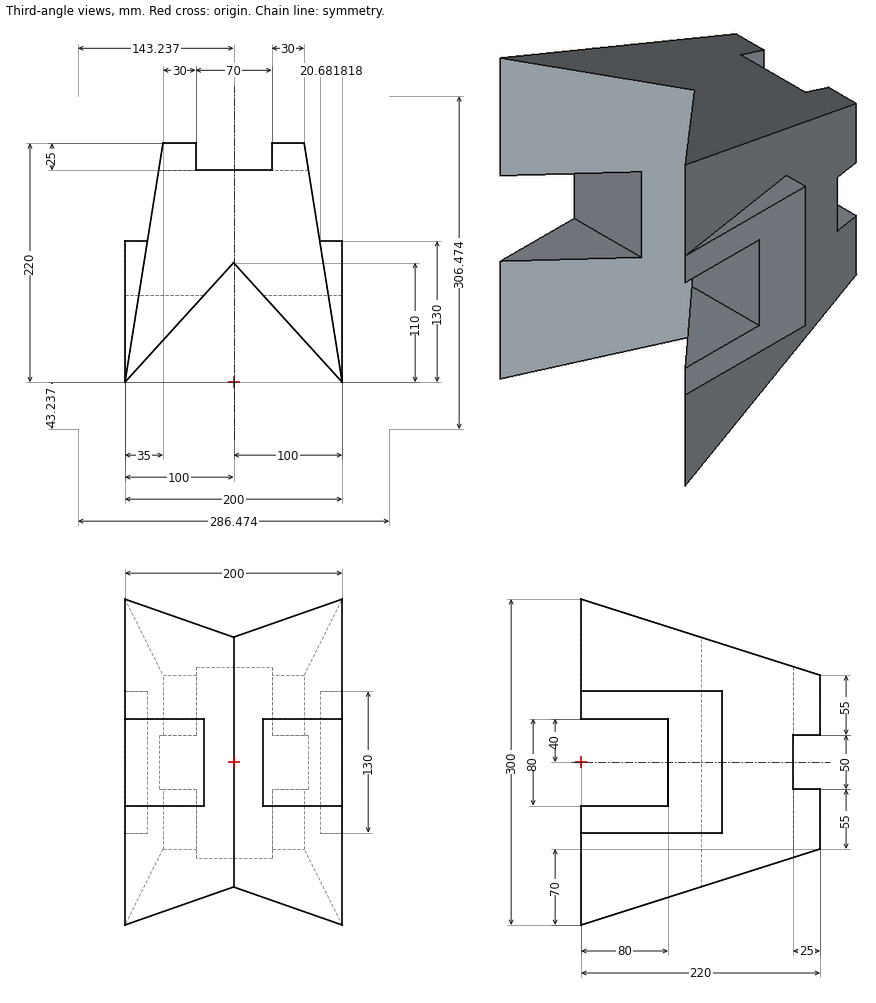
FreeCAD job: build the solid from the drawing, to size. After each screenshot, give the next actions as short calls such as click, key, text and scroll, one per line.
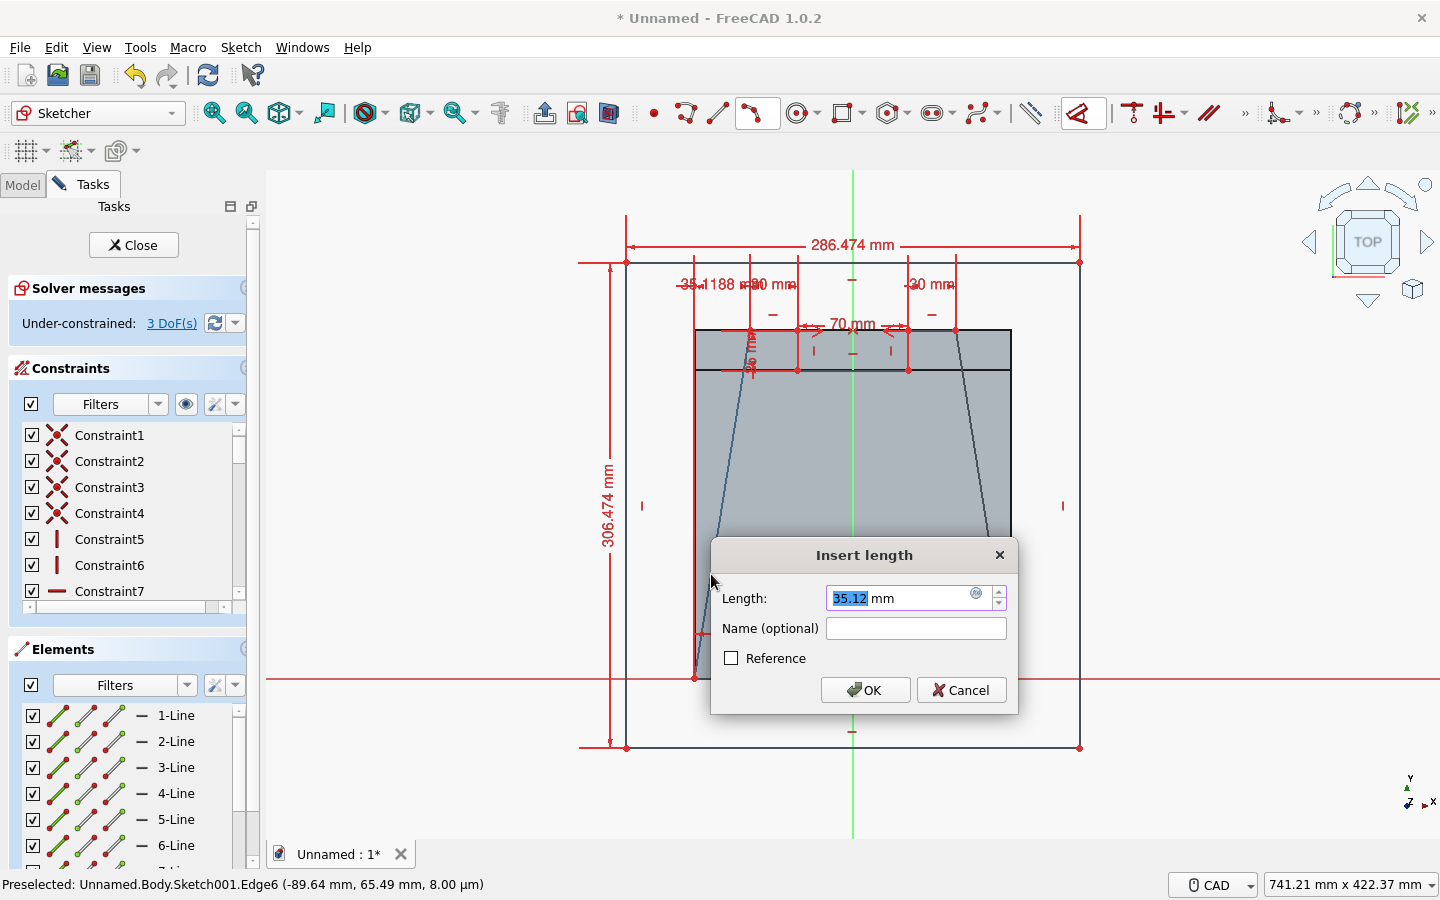
text(35)
key(Return)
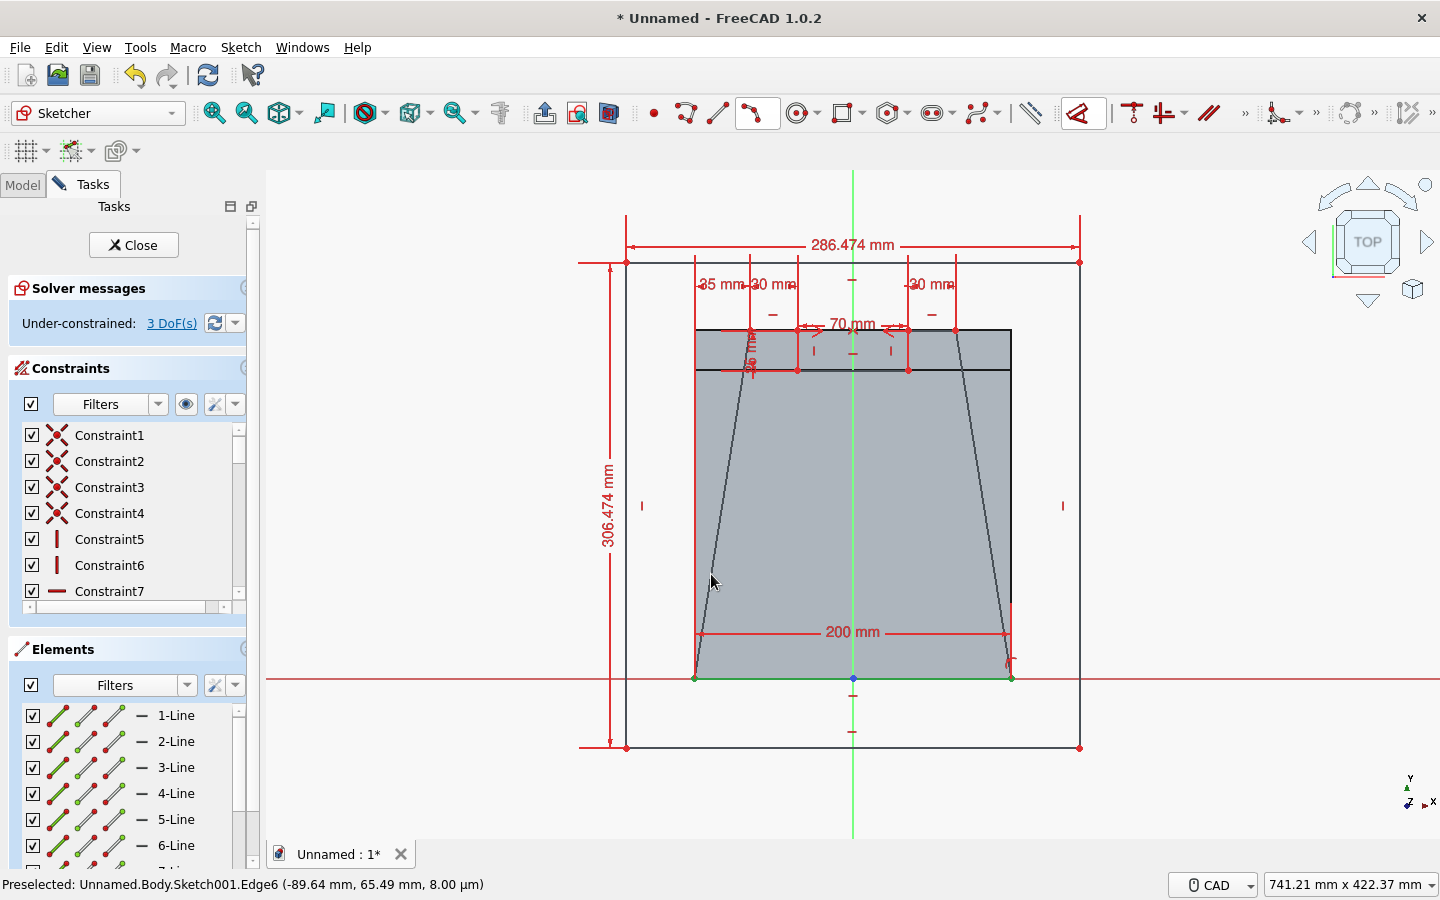
click(750, 331)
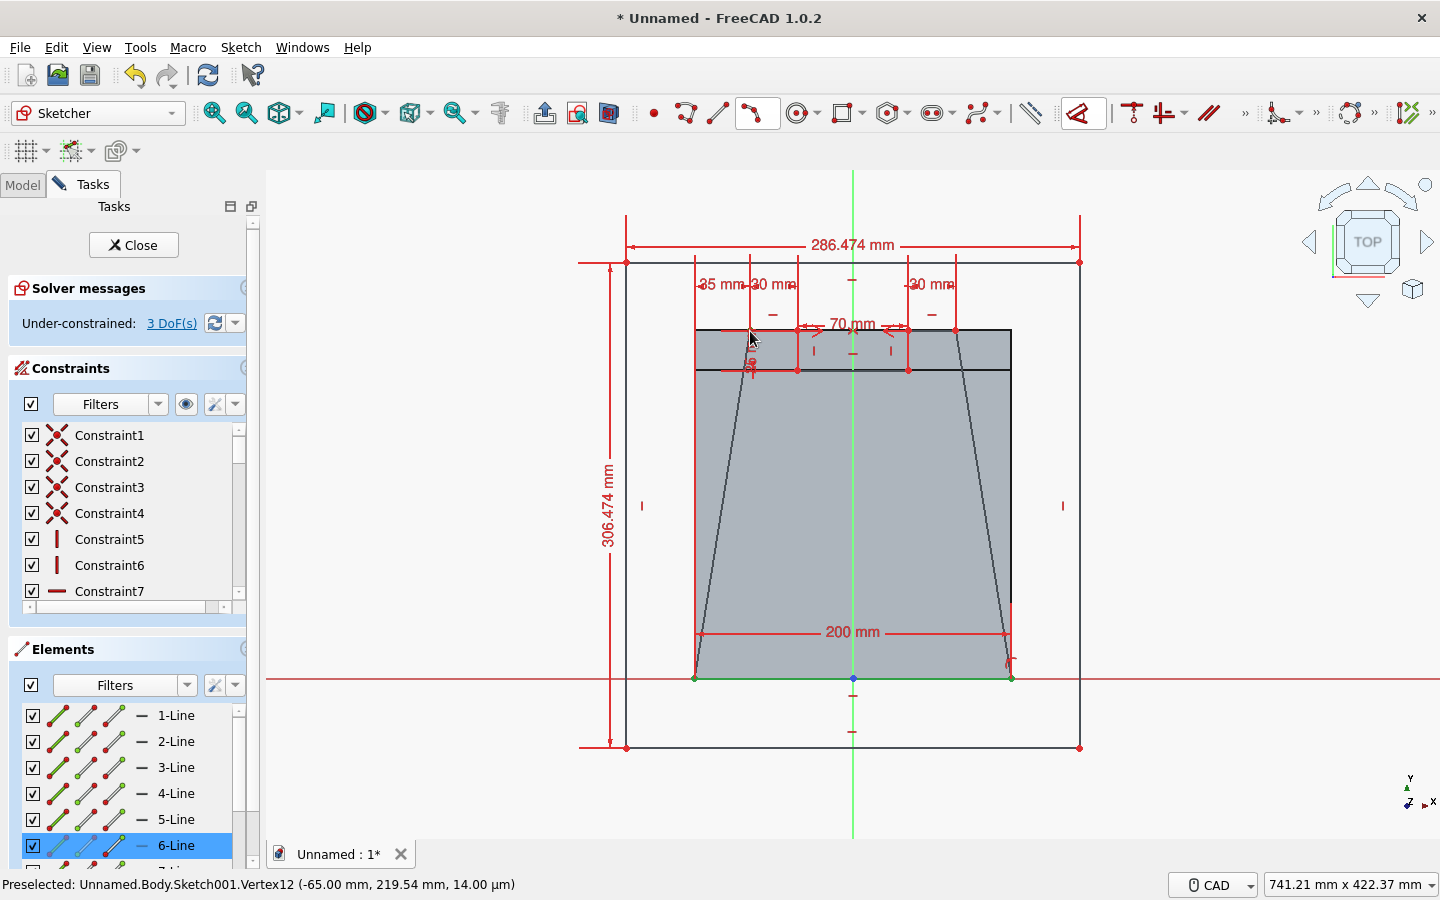
key(i)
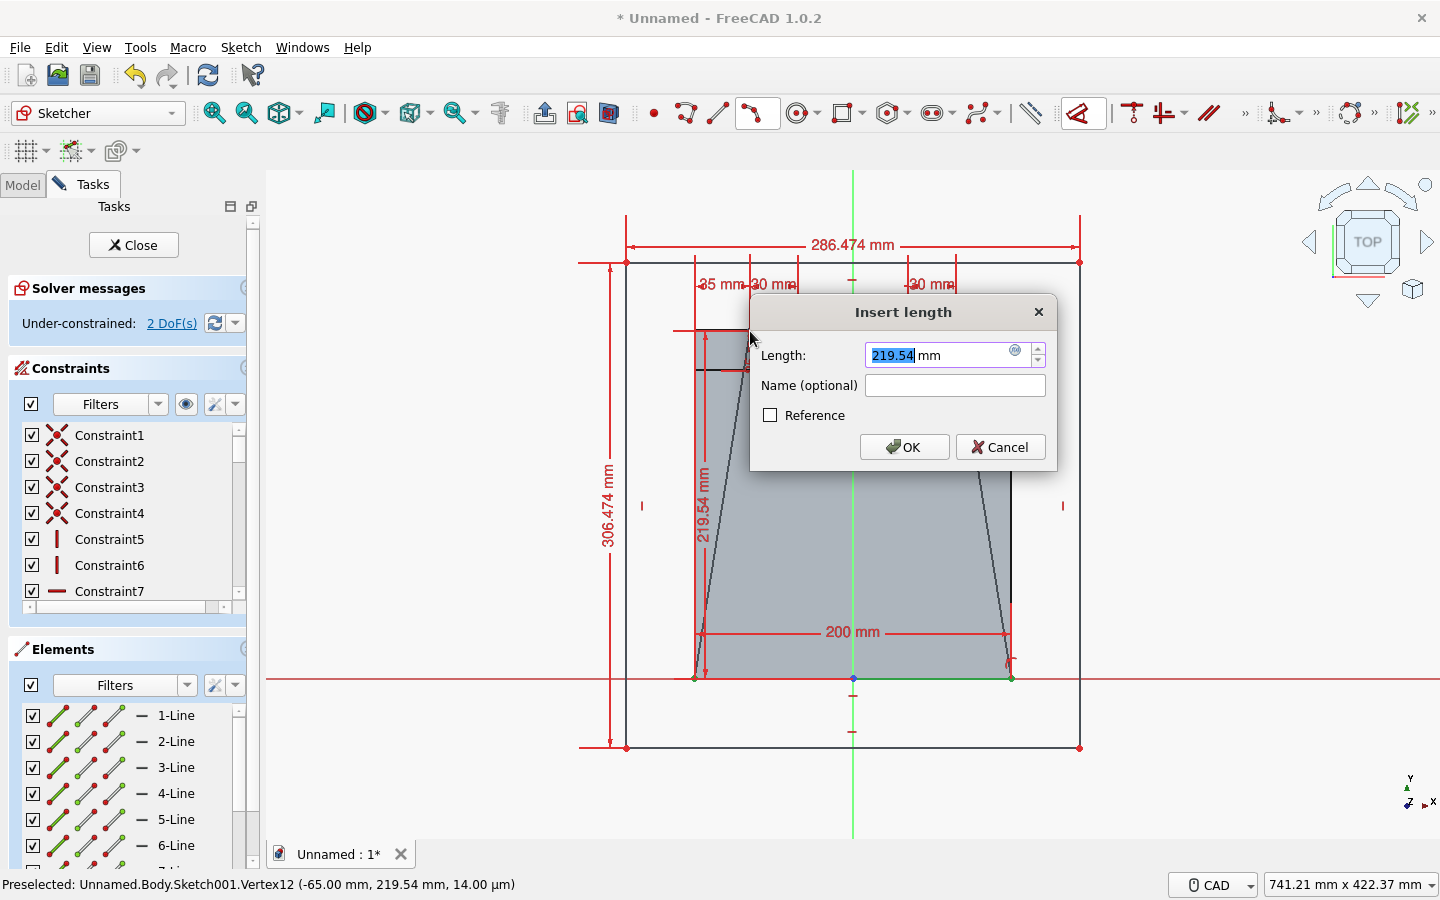
text(220)
key(Return)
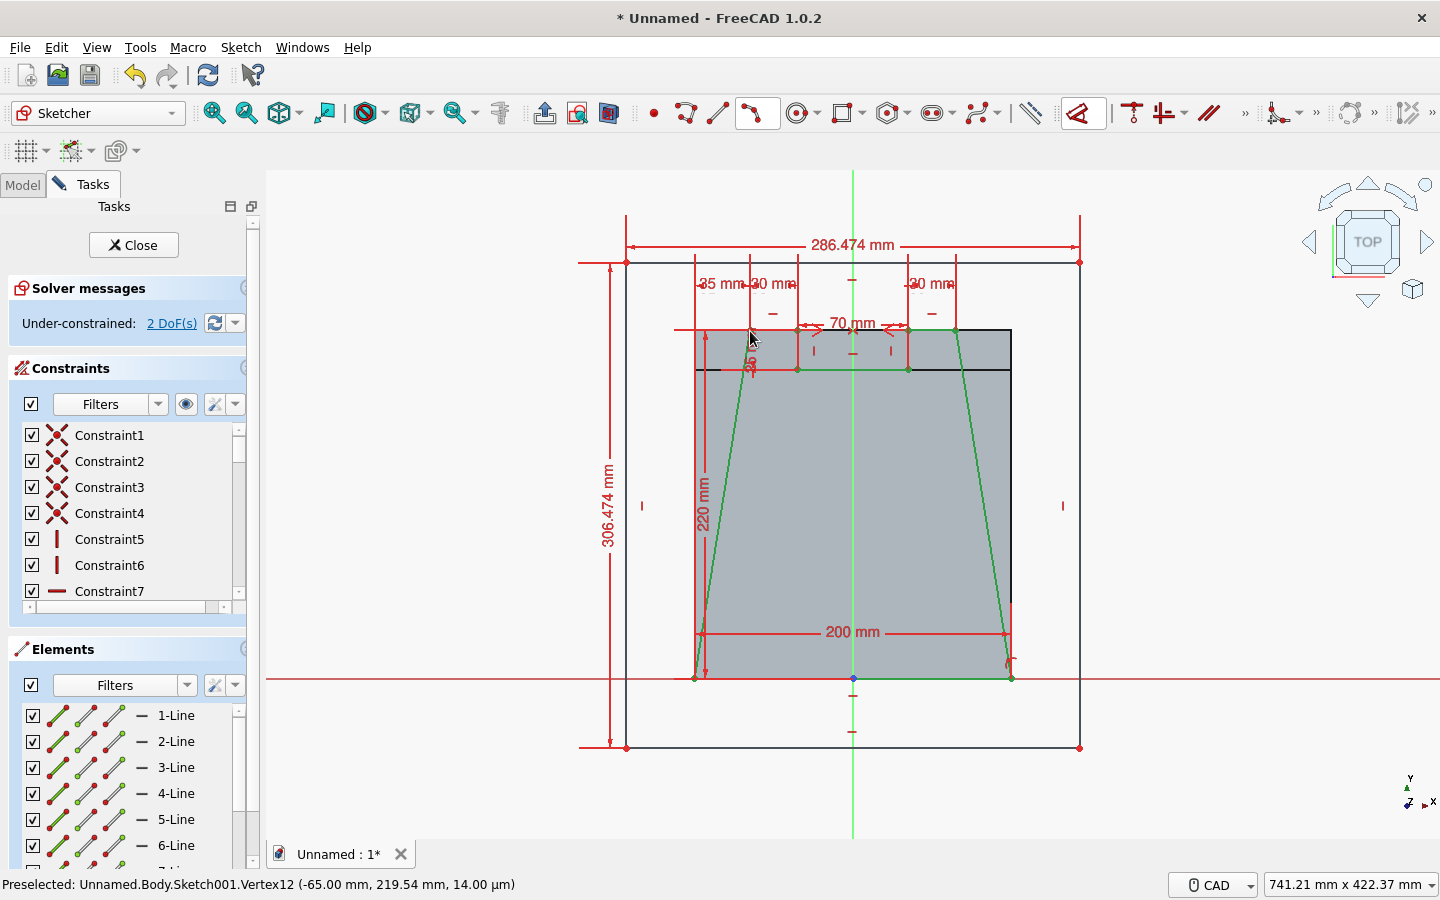
click(626, 748)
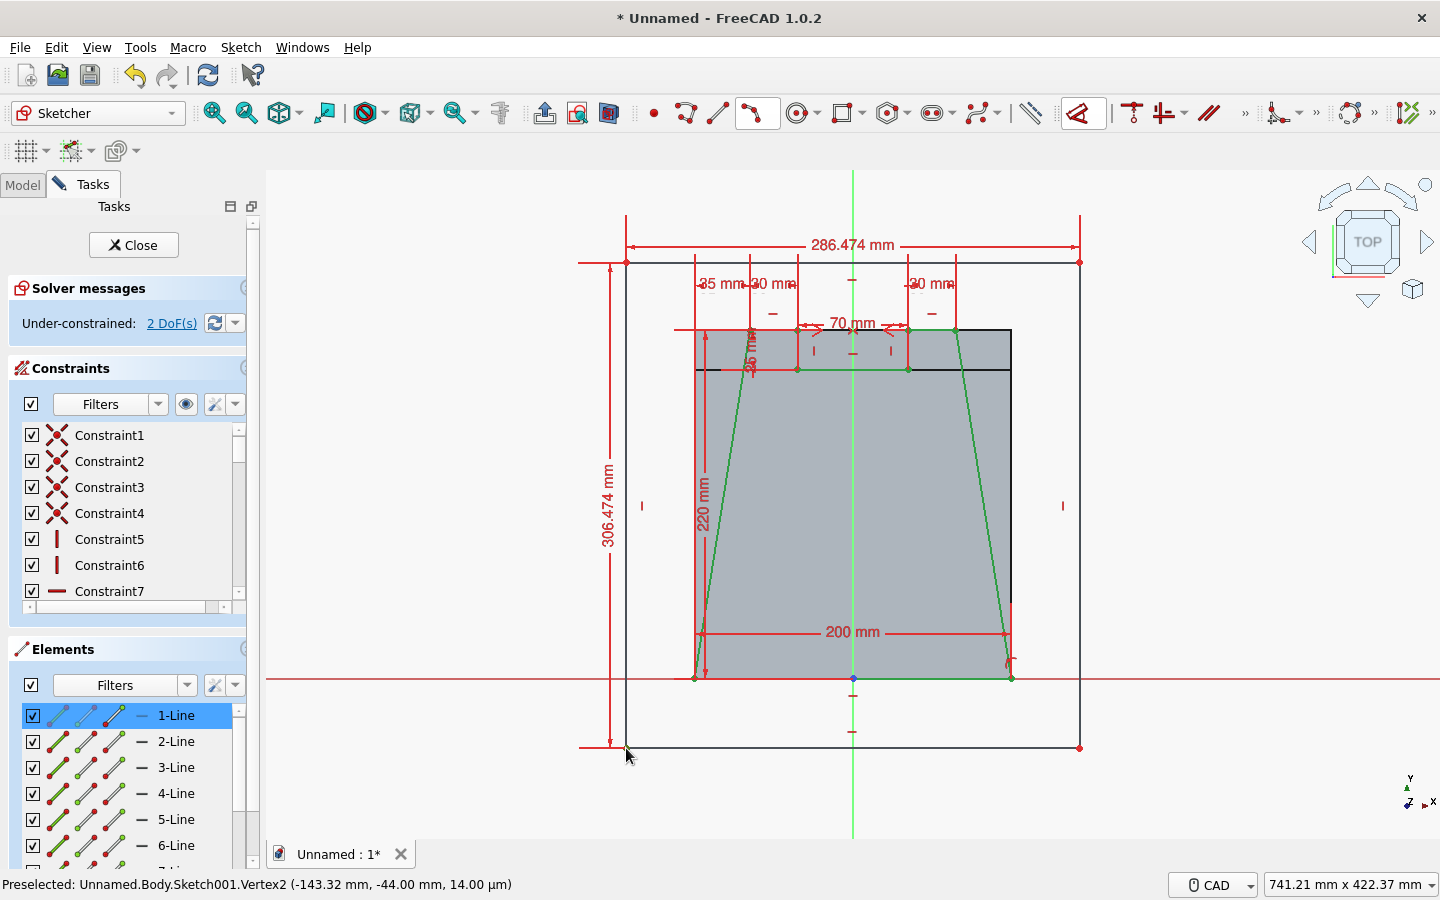
click(1100, 114)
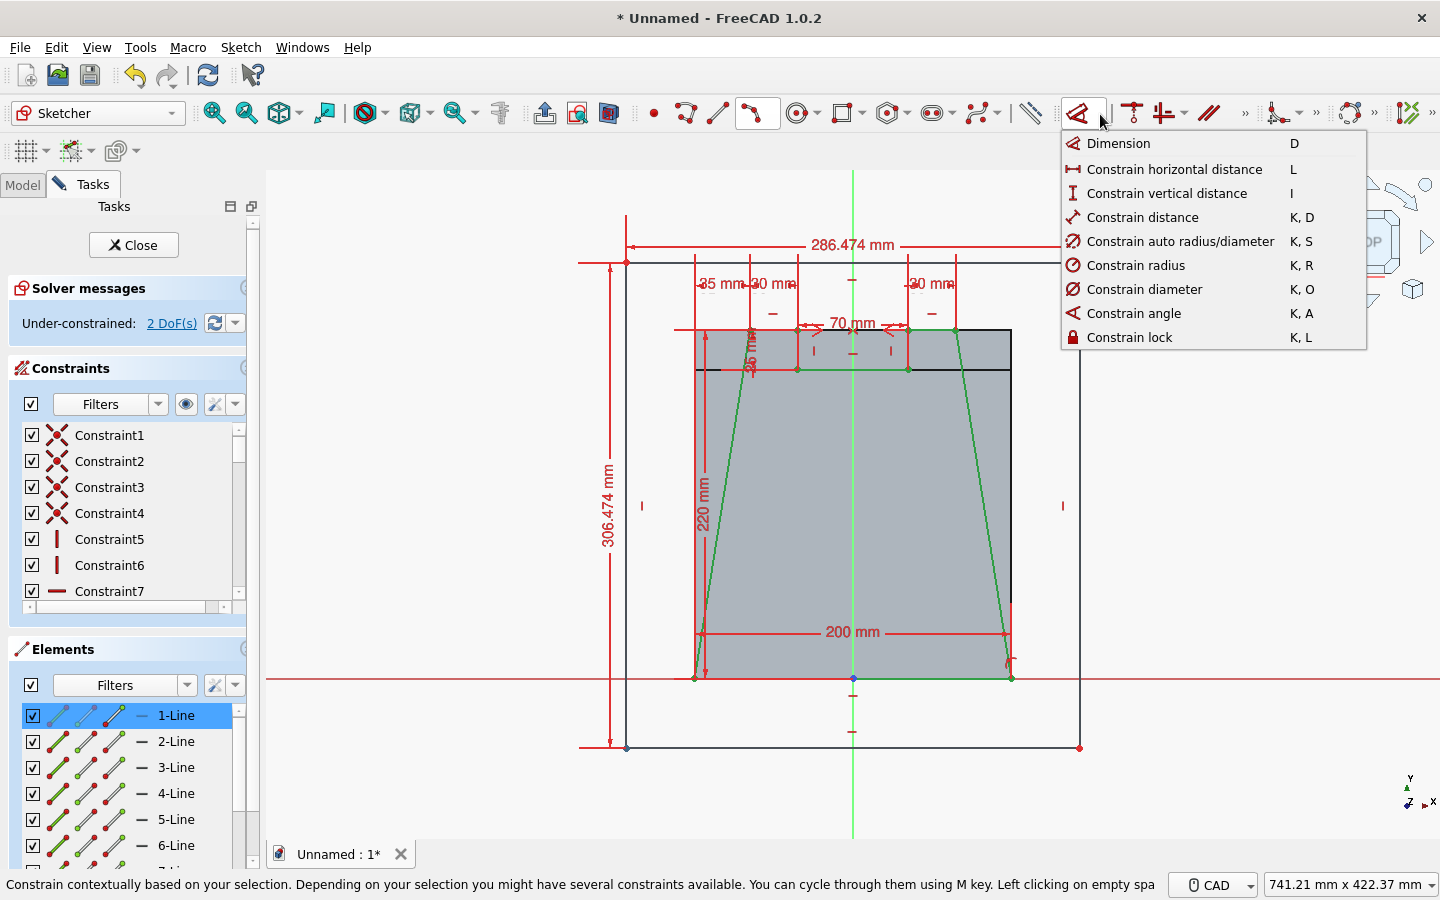
click(1214, 193)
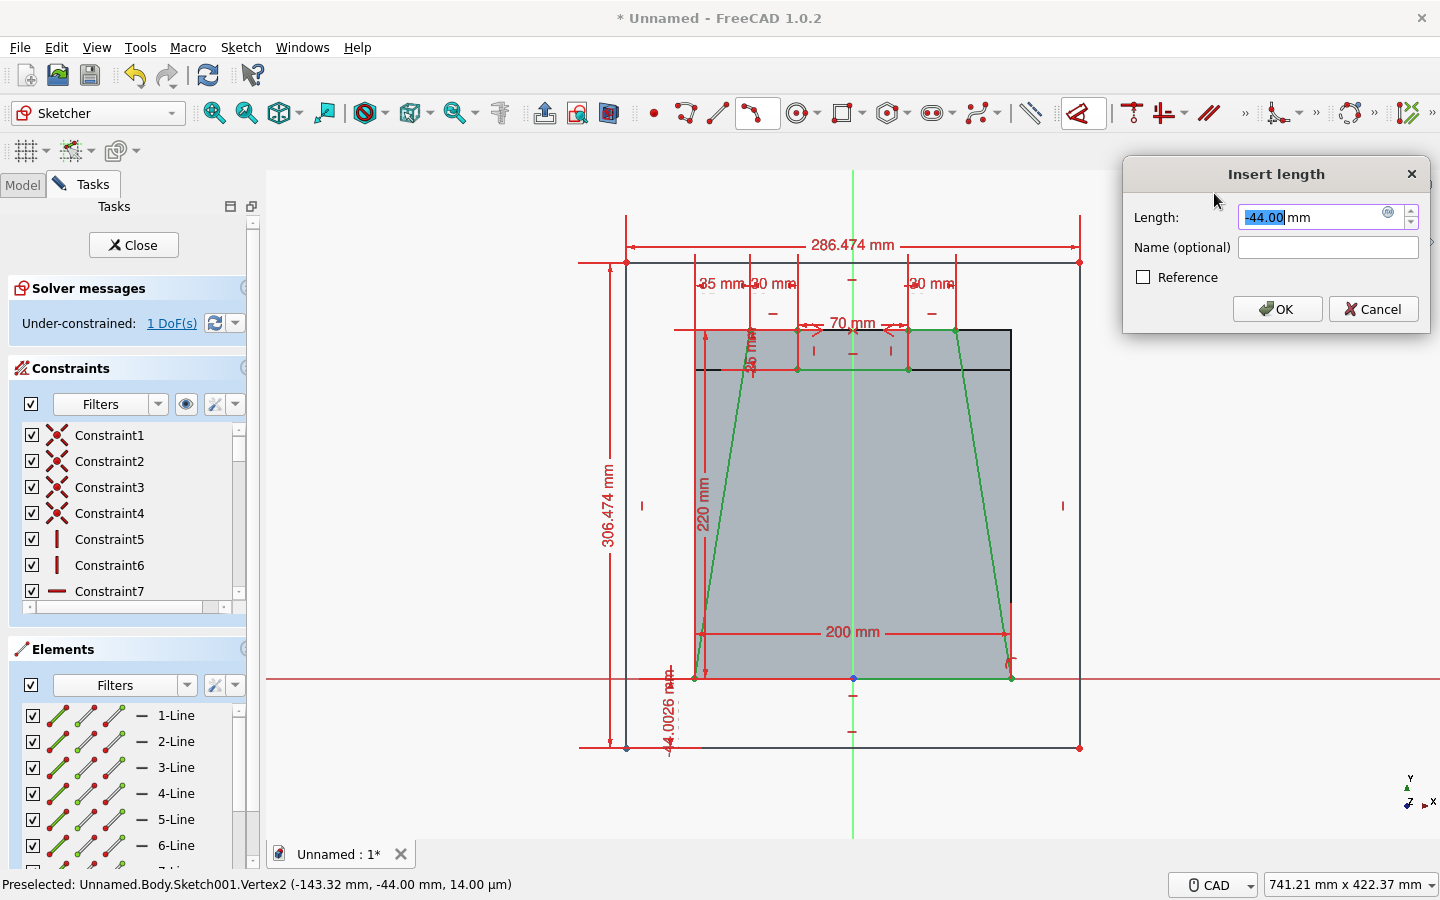
text(-43.237)
key(Return)